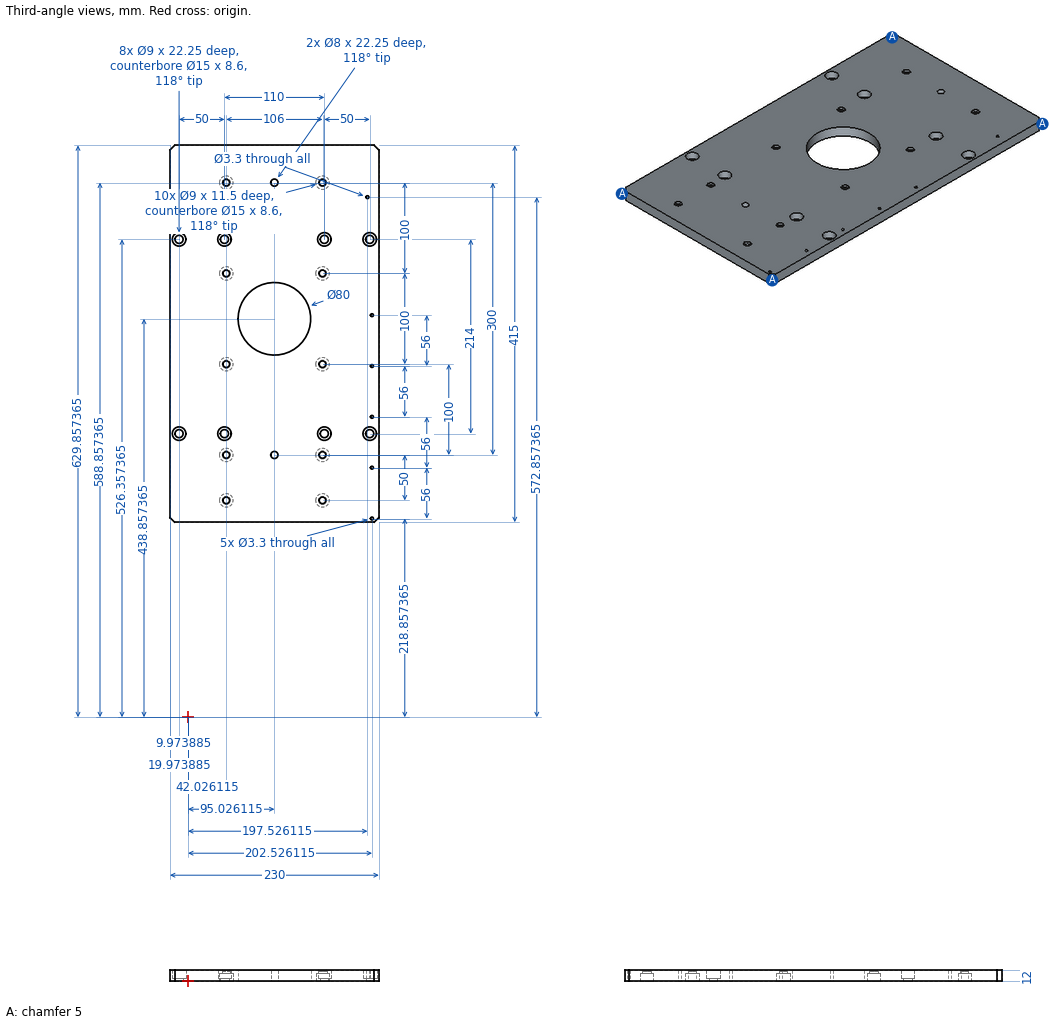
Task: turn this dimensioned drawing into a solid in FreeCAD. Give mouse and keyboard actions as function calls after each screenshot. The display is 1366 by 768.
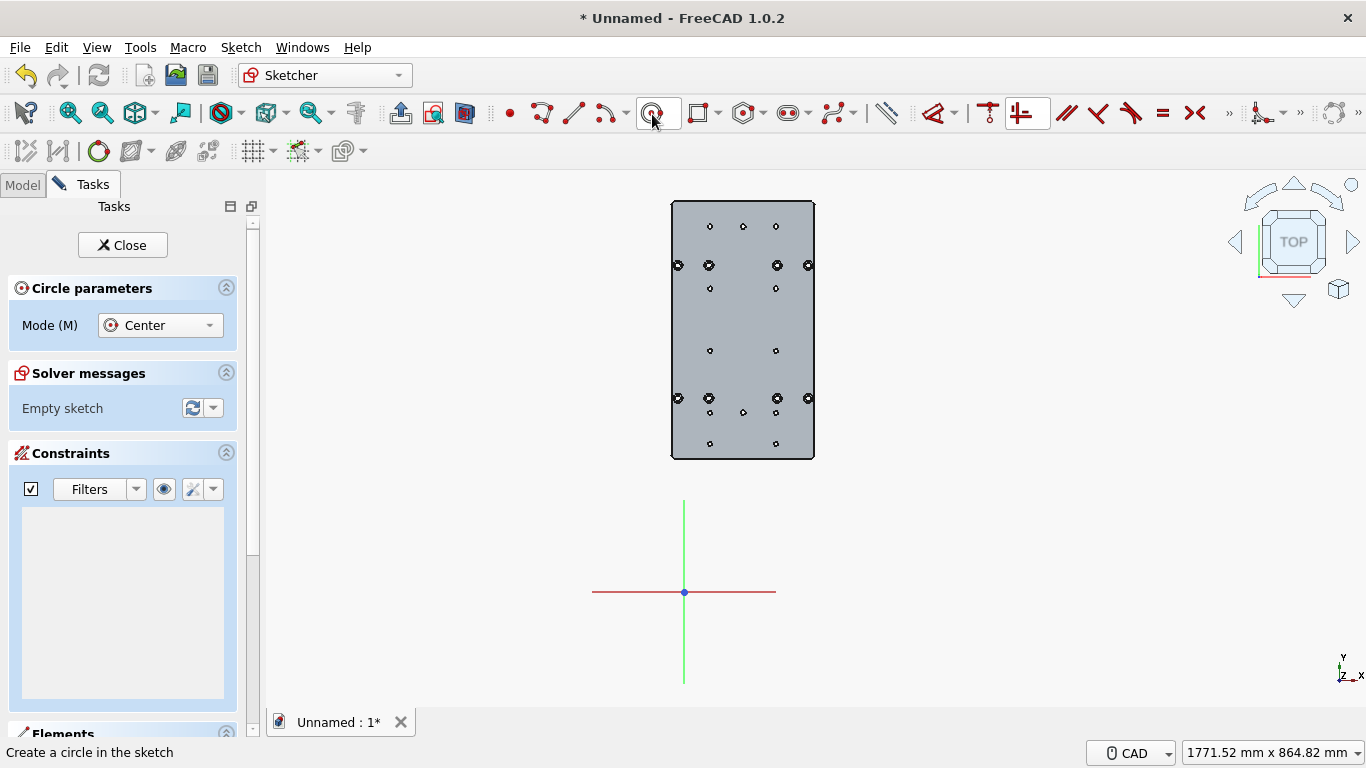
scroll(810, 456, up, 16)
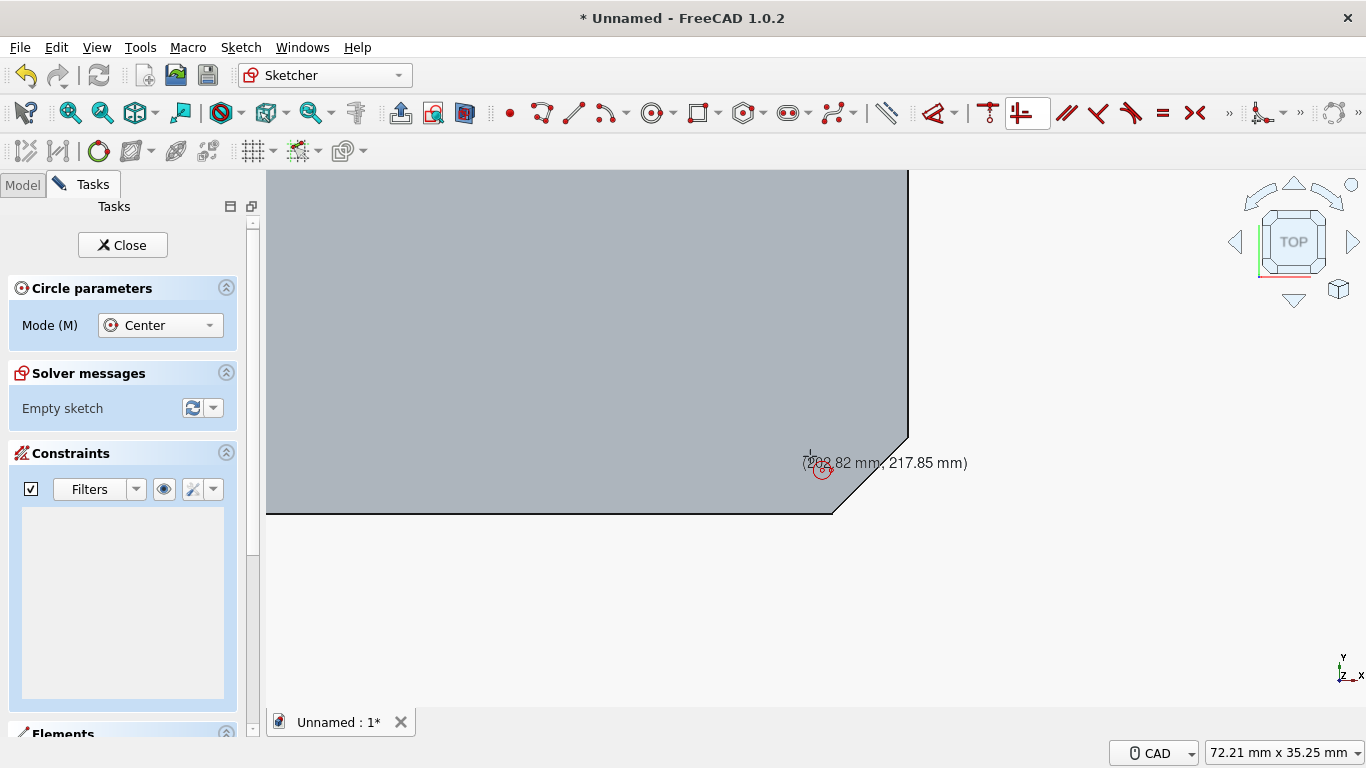
scroll(825, 440, down, 15)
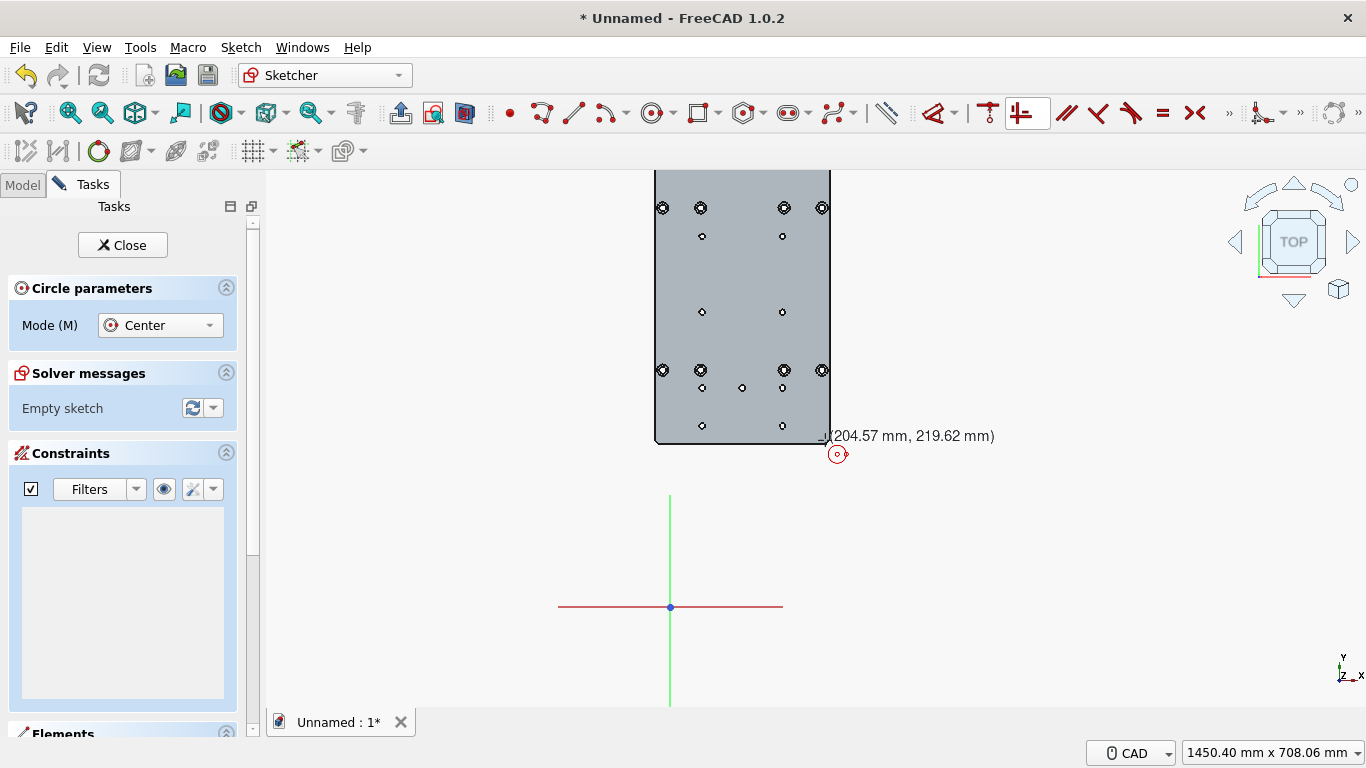
click(824, 441)
move(825, 440)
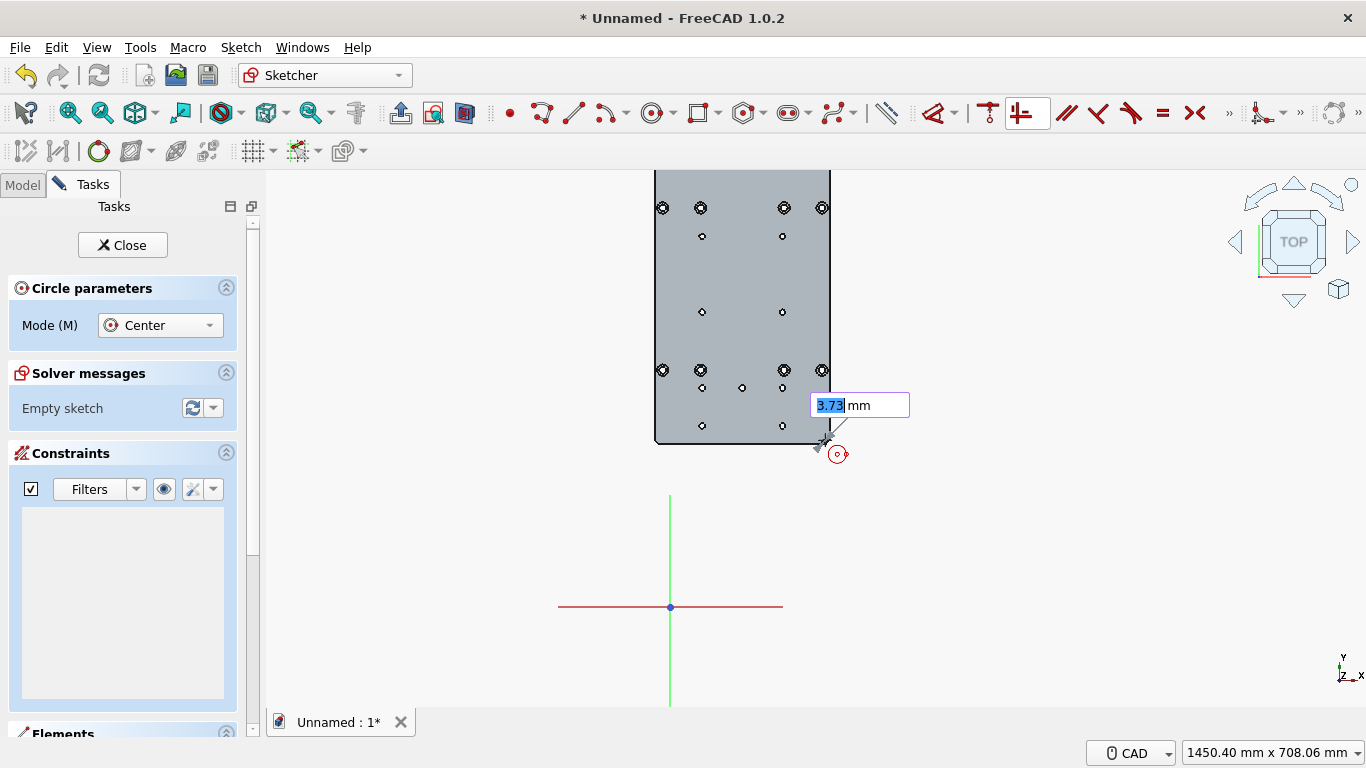
text(3.3)
key(Return)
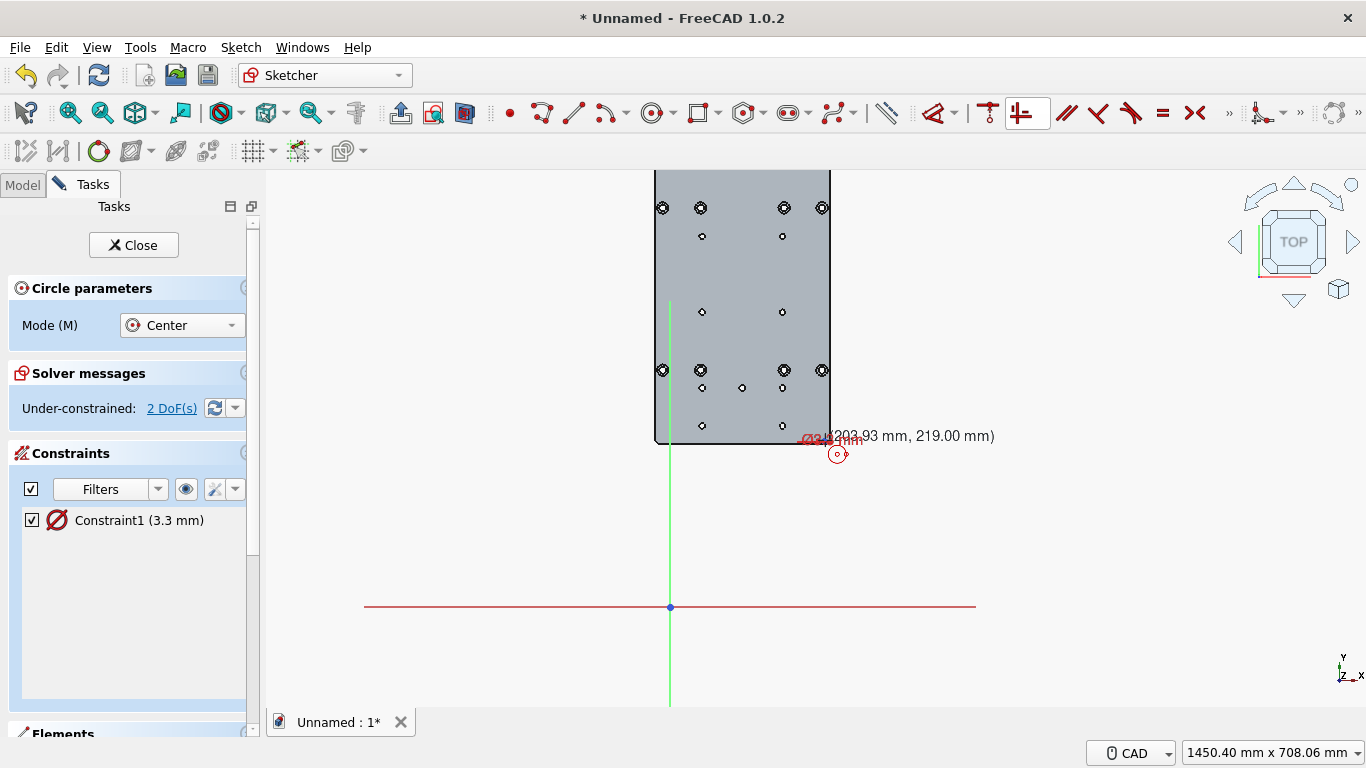
scroll(824, 399, up, 15)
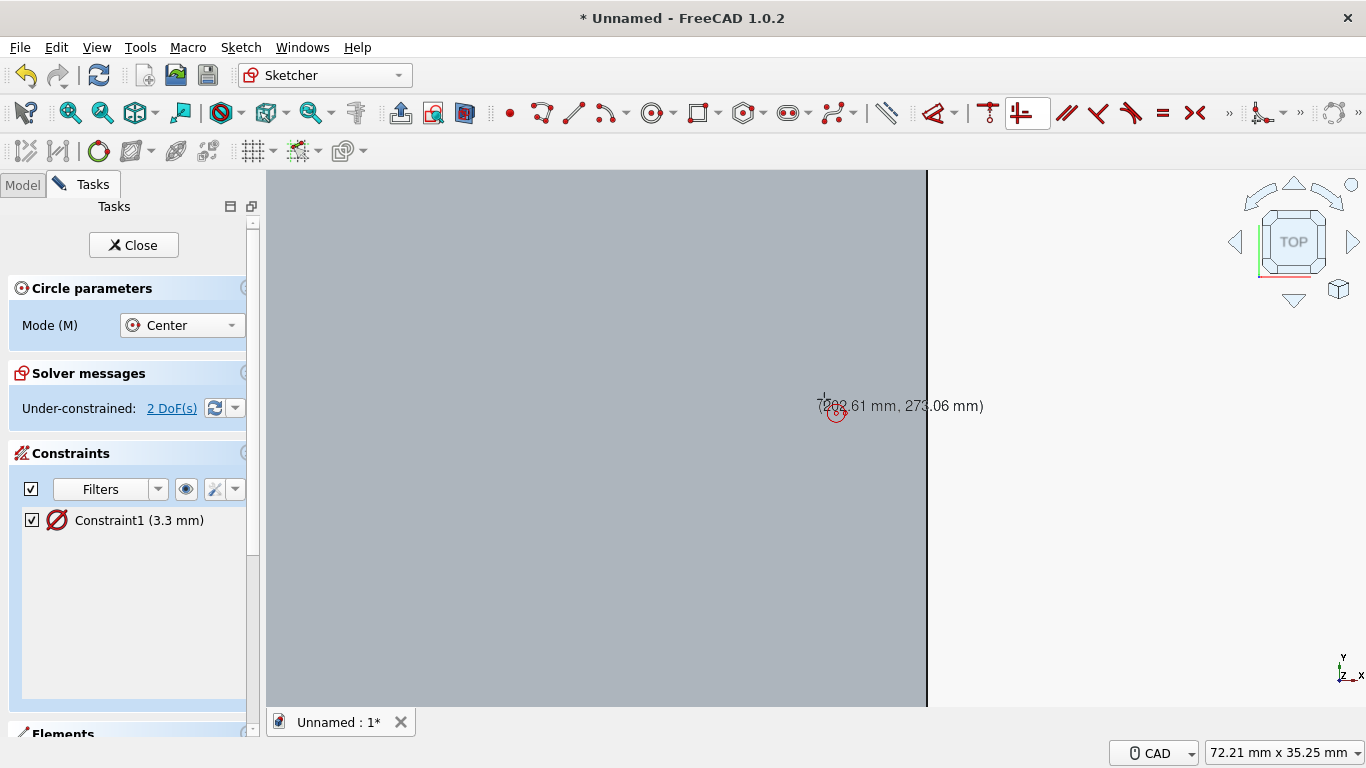
scroll(824, 399, down, 15)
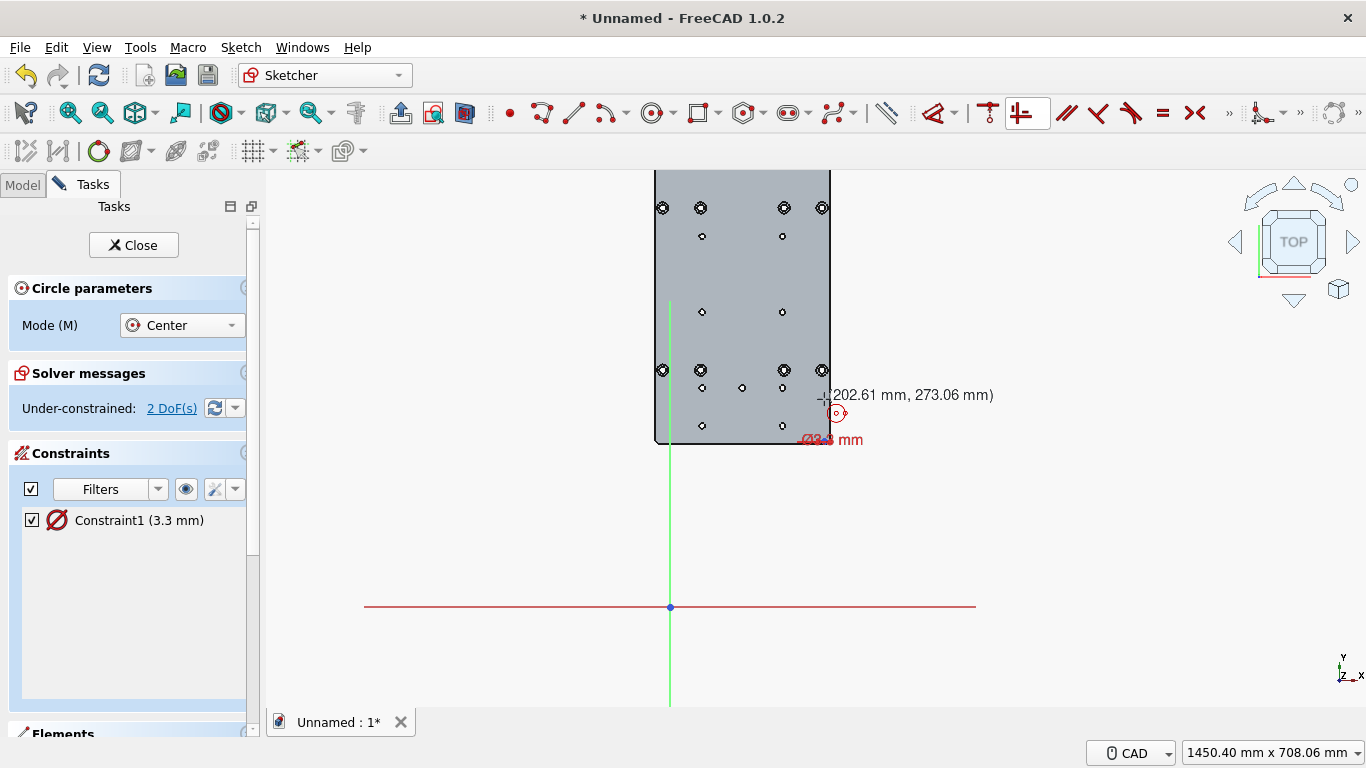
click(824, 399)
move(825, 398)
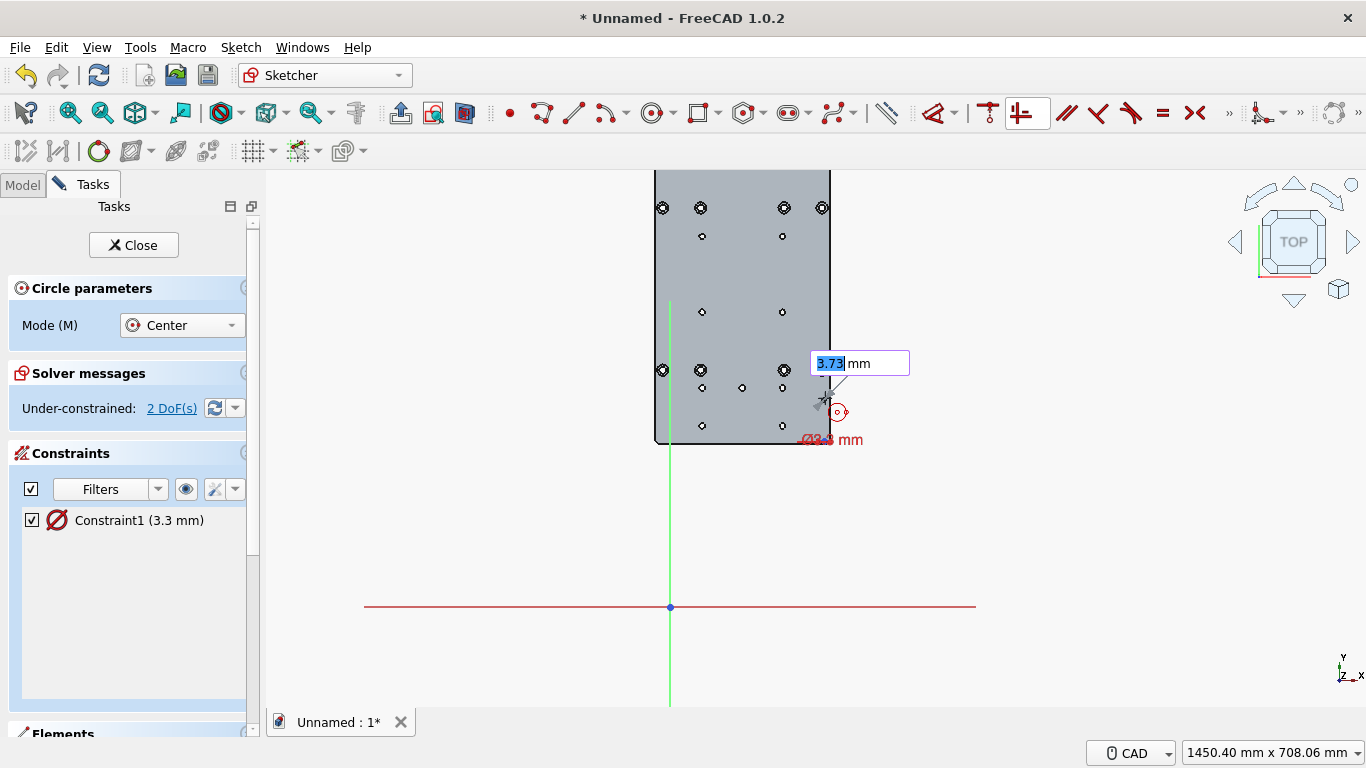
text(3.3)
key(Return)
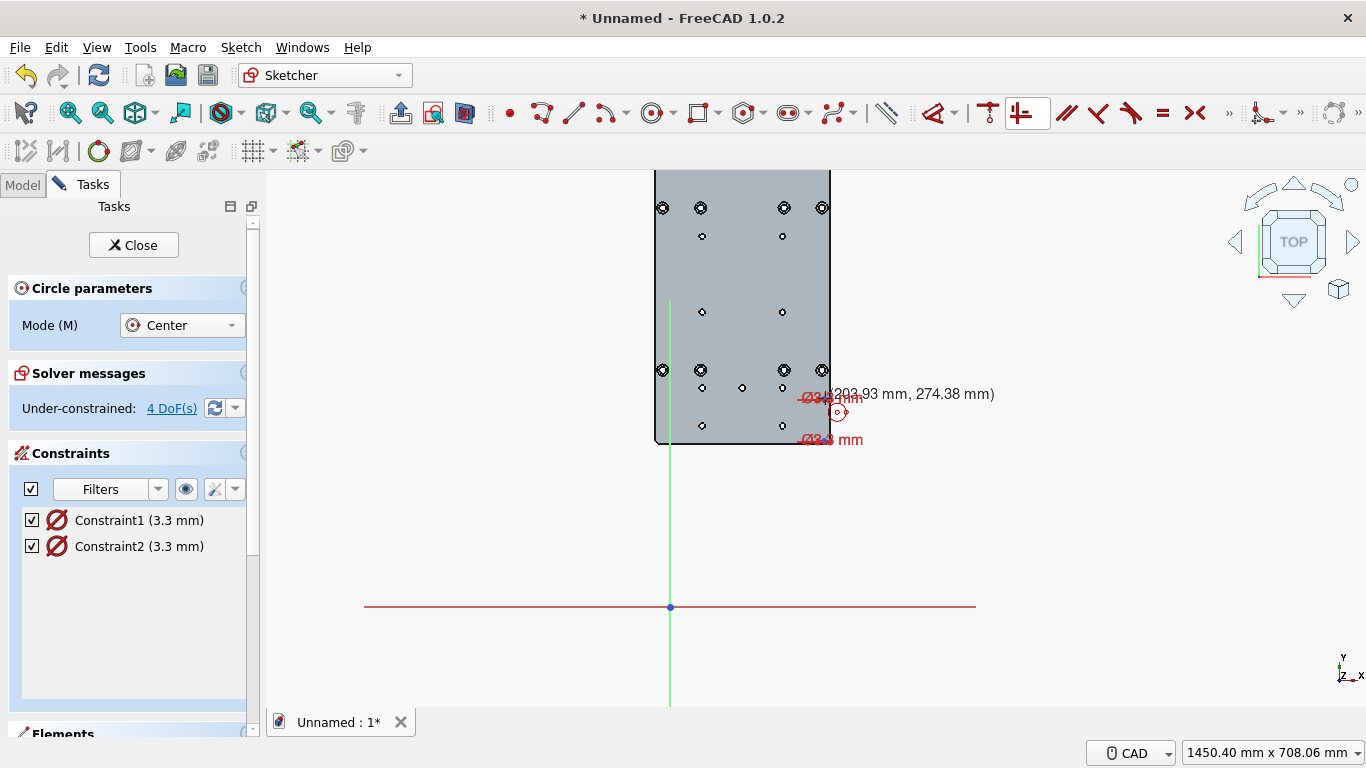
scroll(824, 356, up, 15)